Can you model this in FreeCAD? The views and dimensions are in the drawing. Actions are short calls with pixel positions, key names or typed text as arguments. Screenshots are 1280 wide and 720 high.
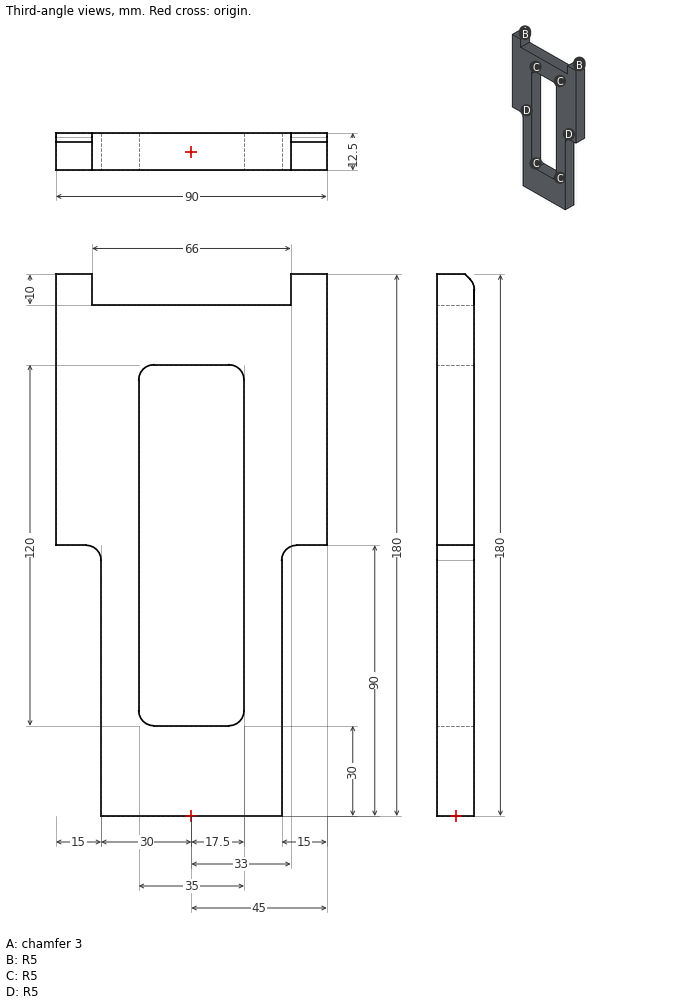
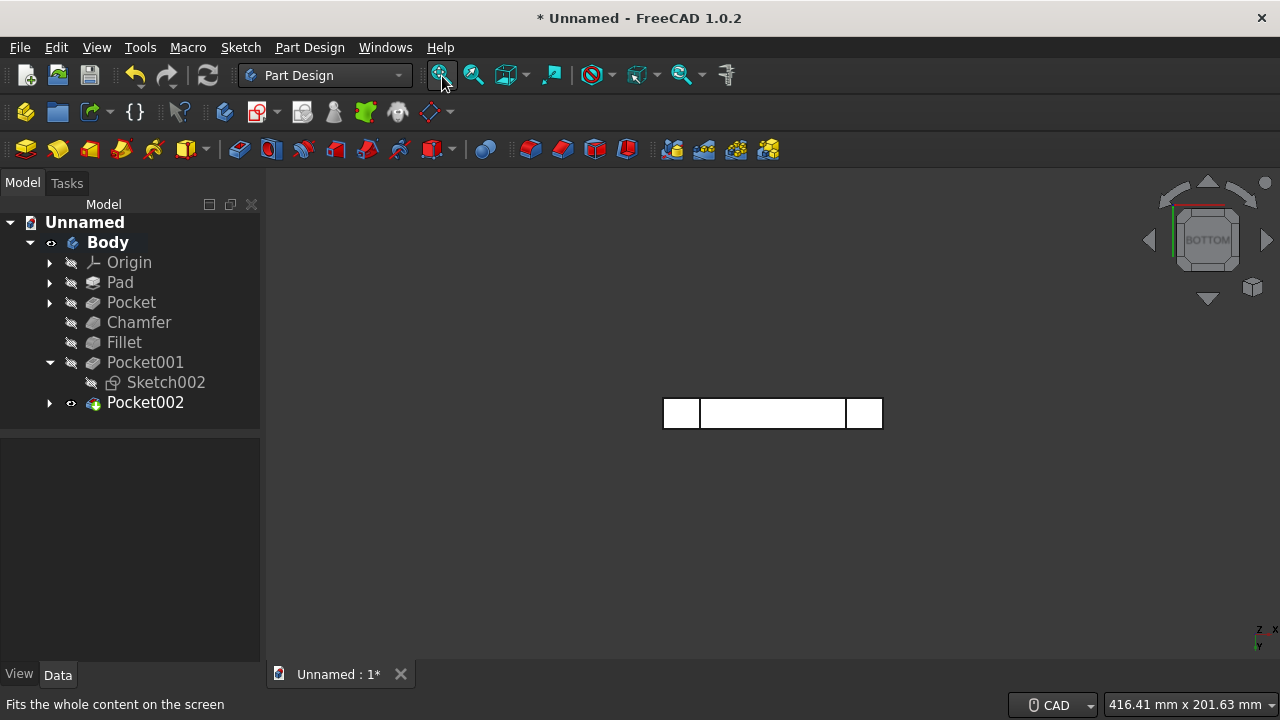
click(442, 76)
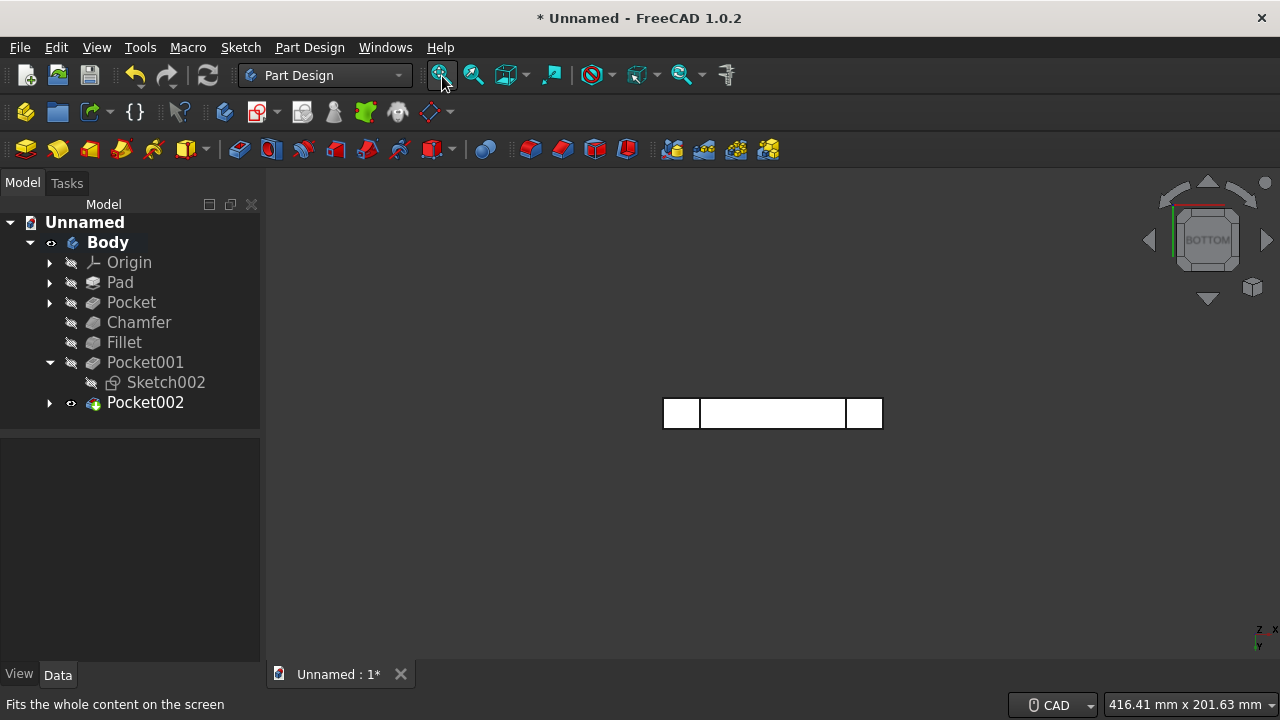
key(4)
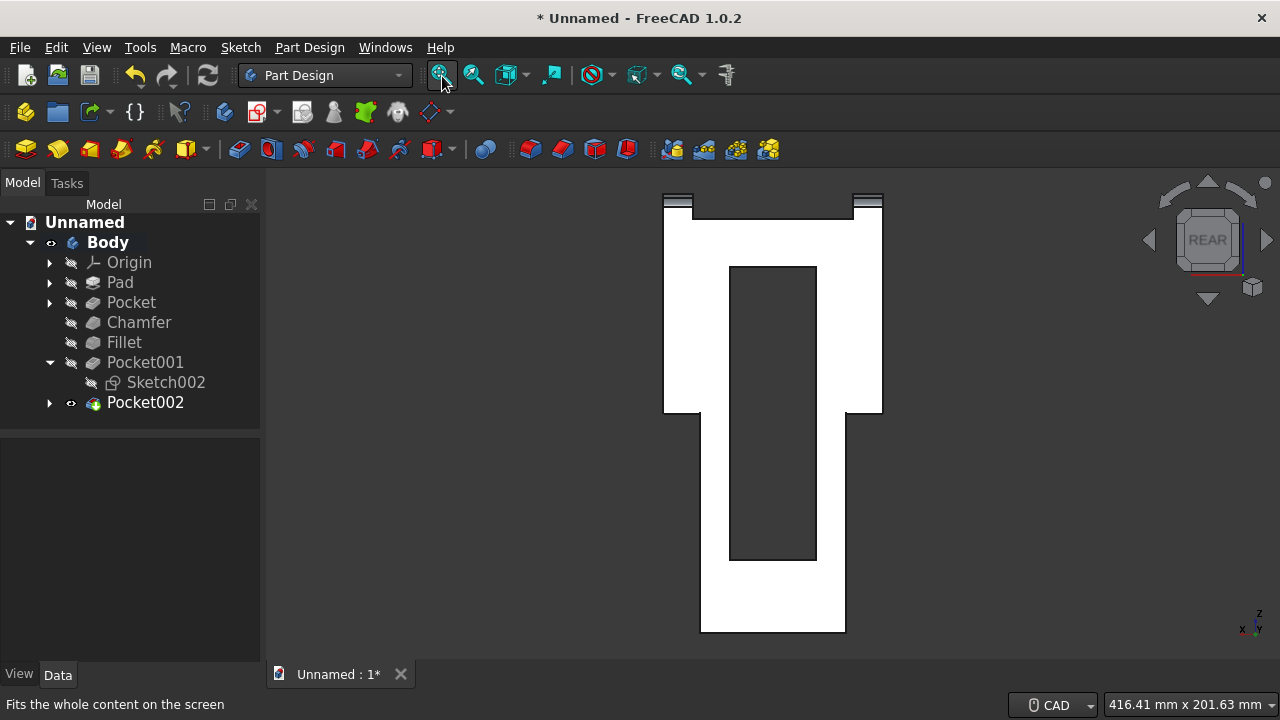
key(6)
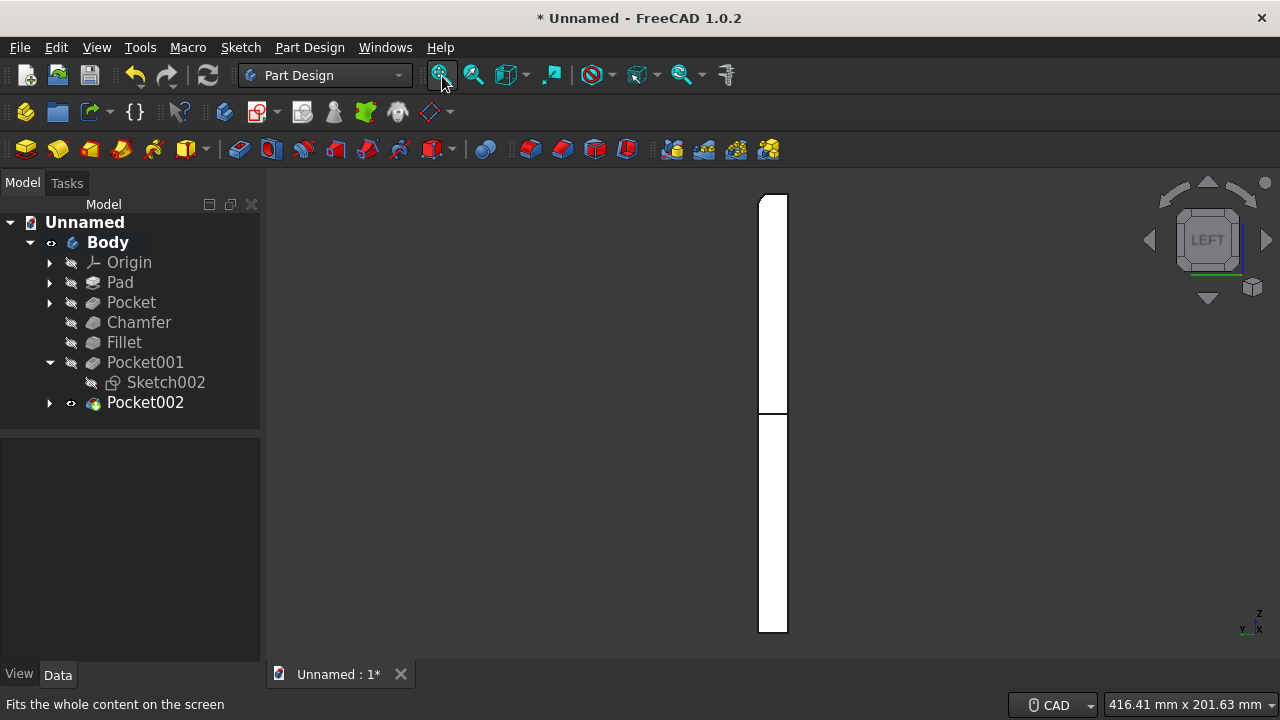
key(v)
key(3)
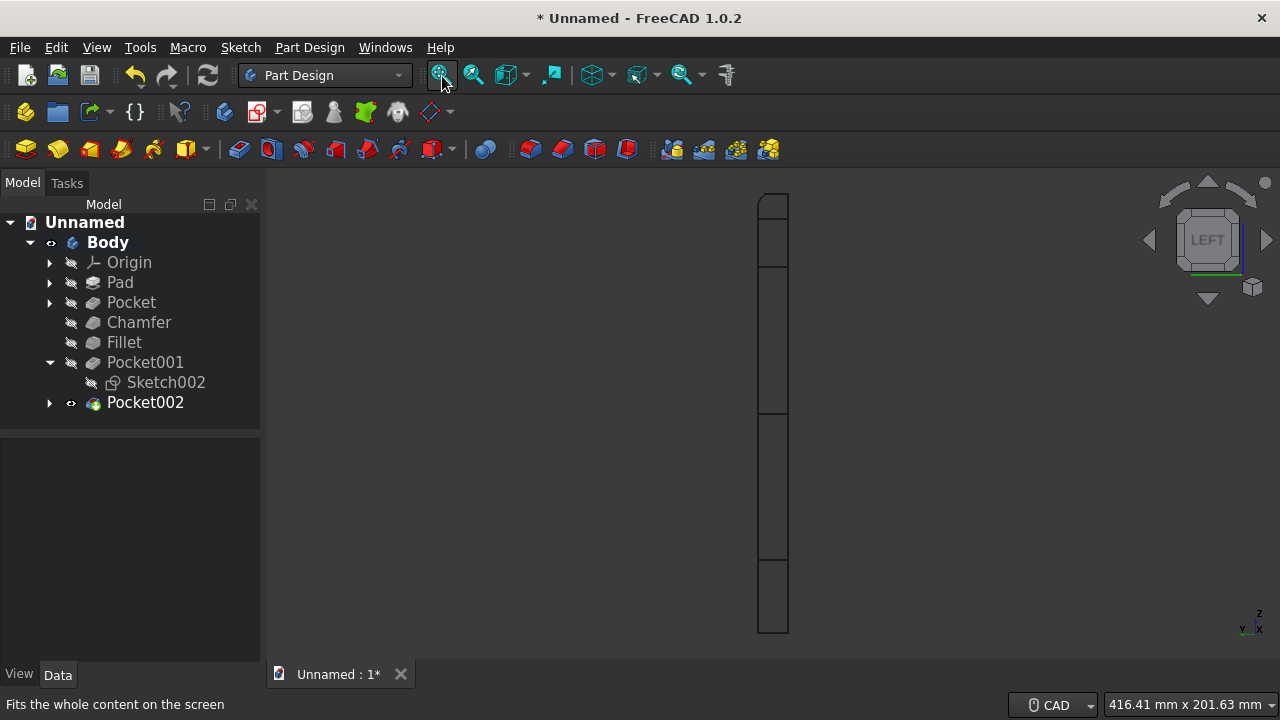
key(0)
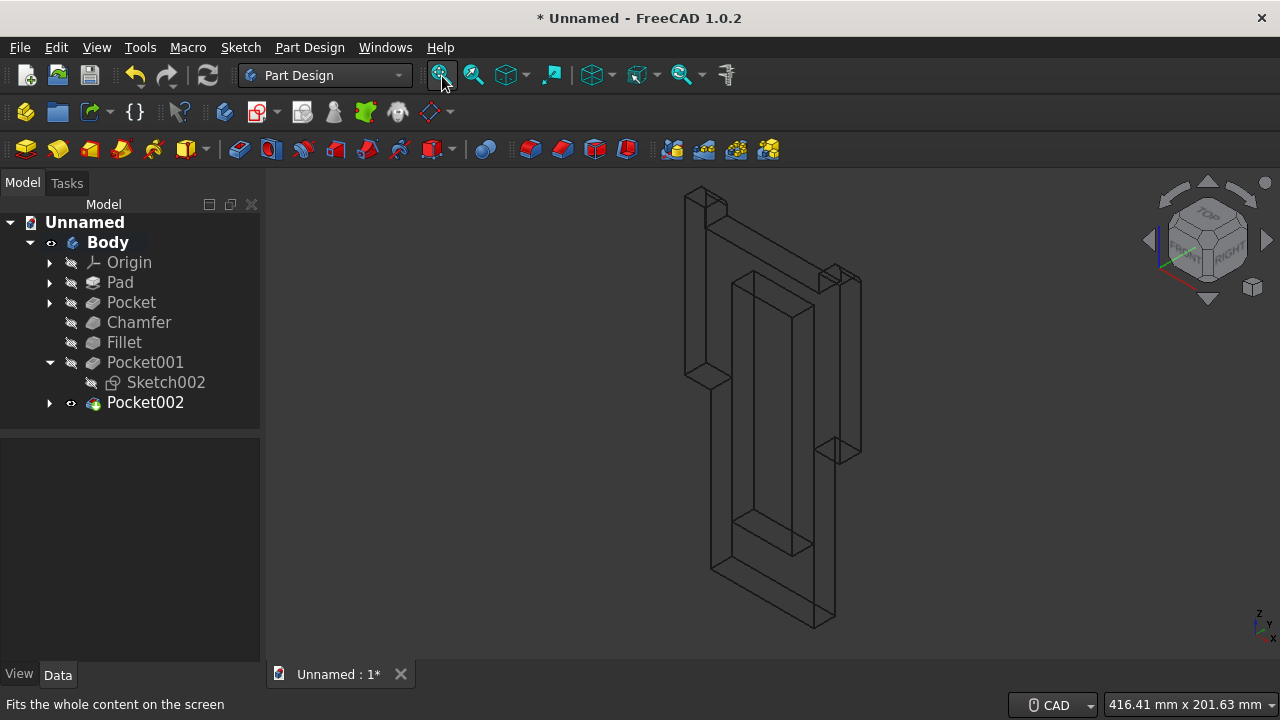
click(743, 276)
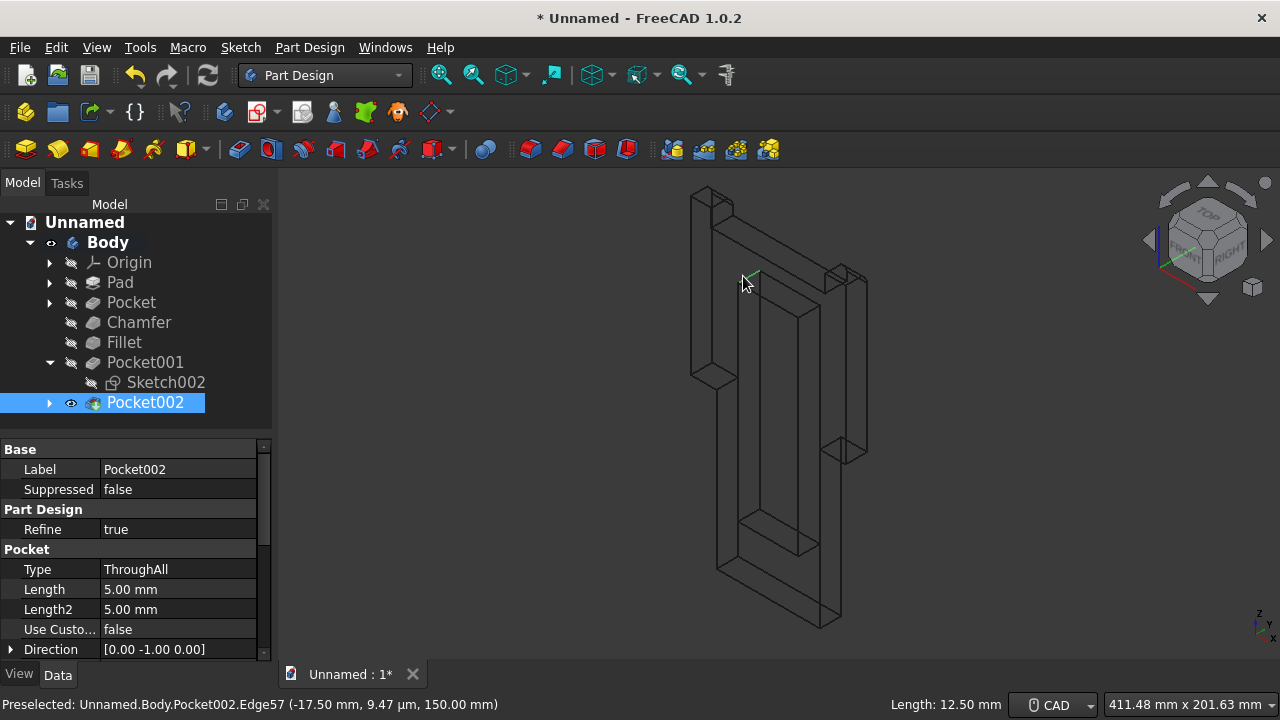
click(749, 514, ctrl)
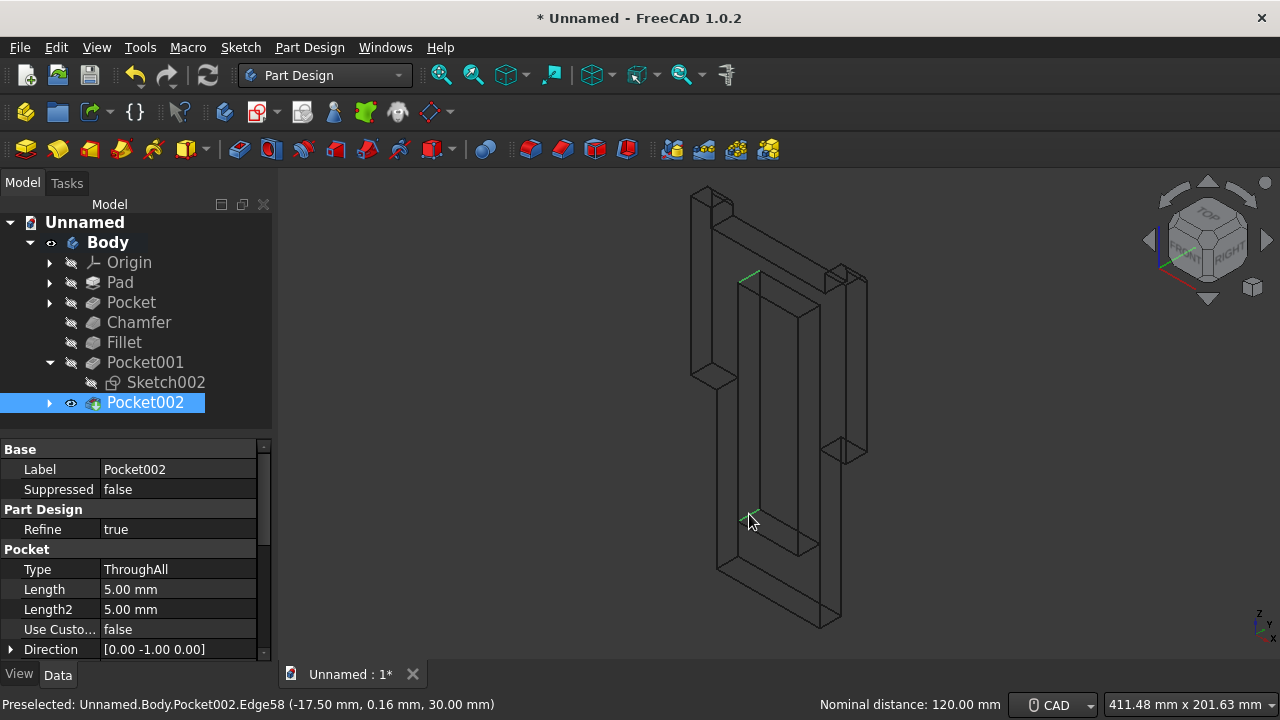
click(809, 549, ctrl)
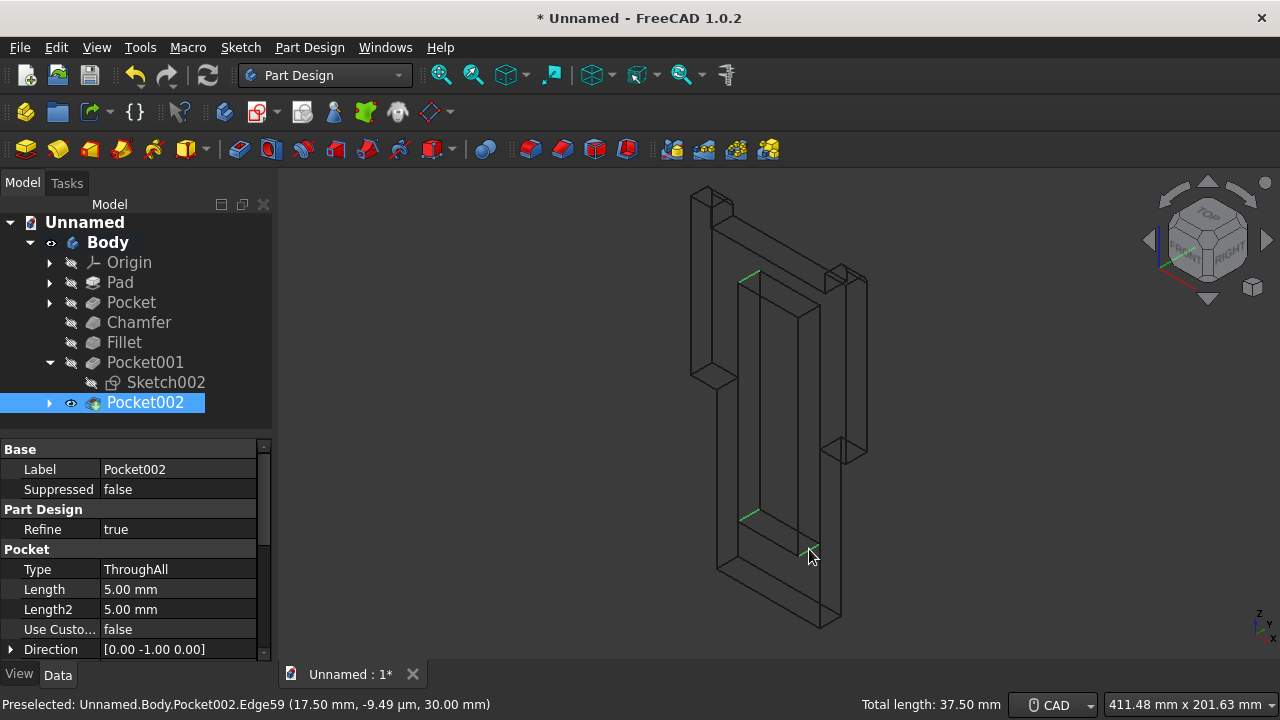
click(809, 311, ctrl)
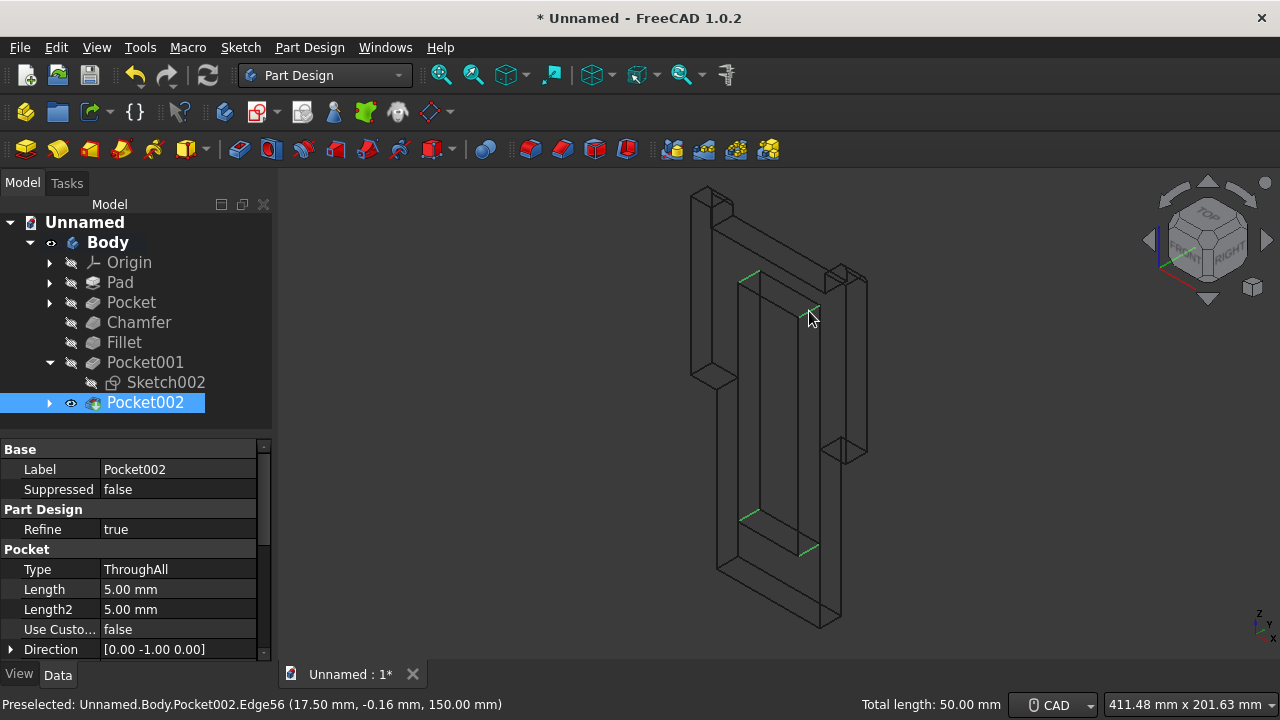
key(v)
key(1)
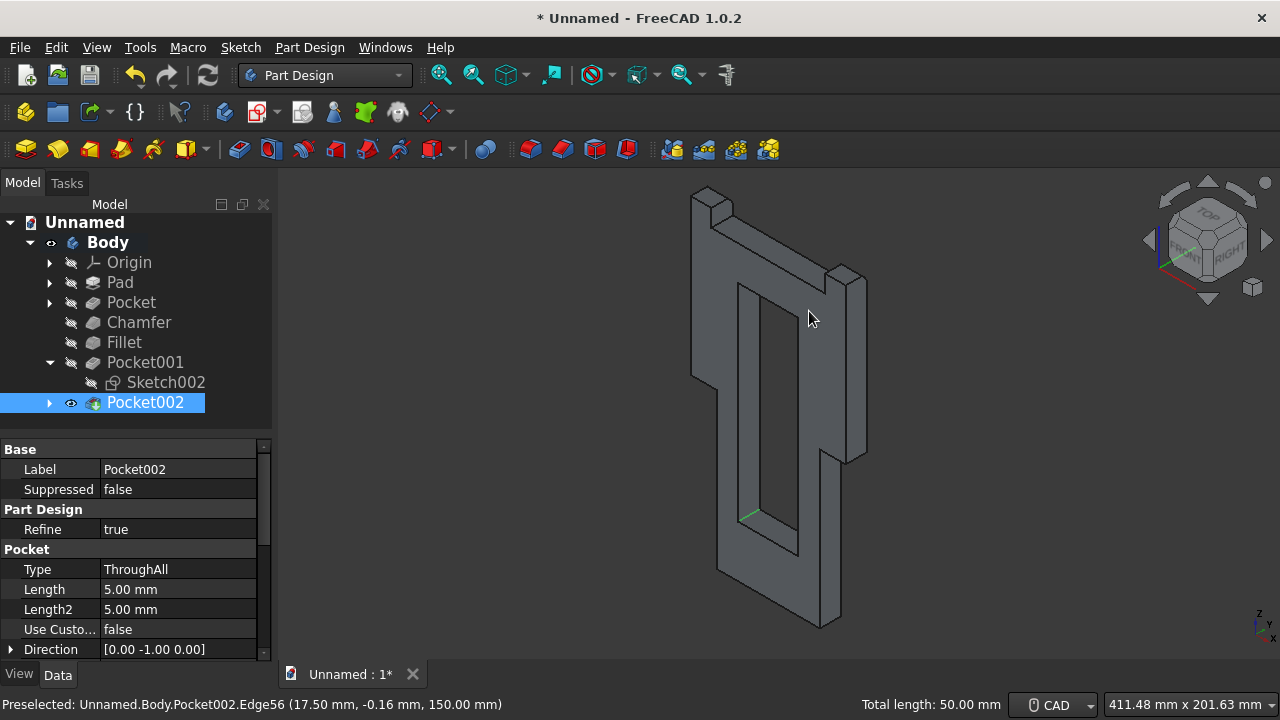
click(532, 150)